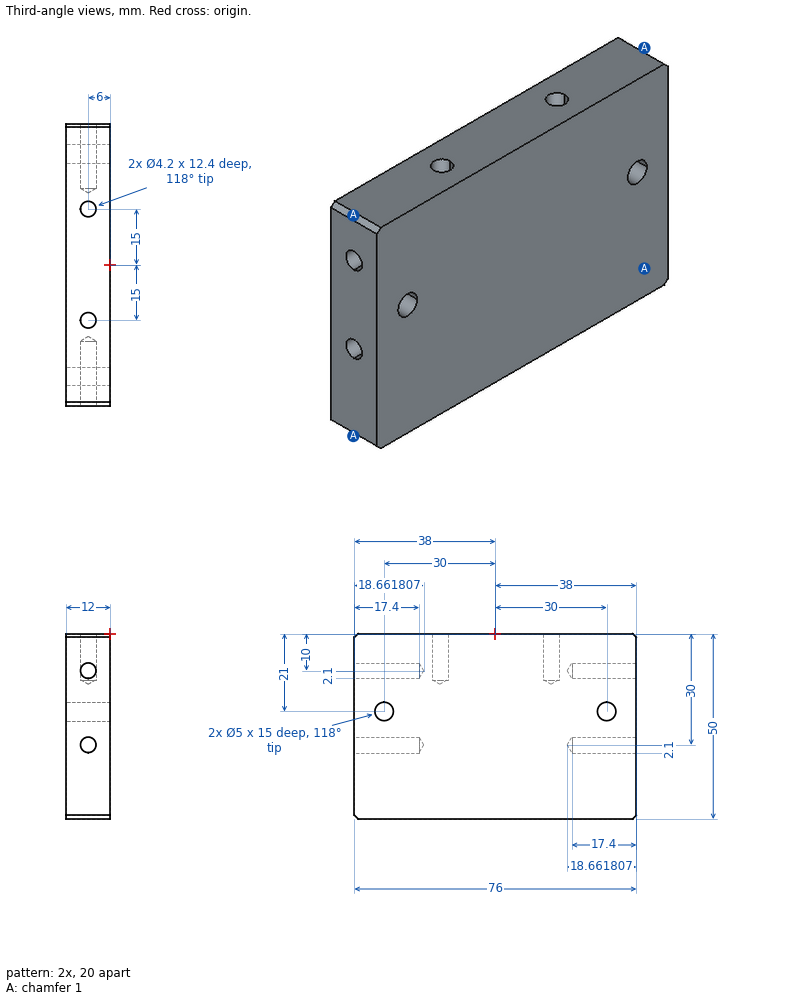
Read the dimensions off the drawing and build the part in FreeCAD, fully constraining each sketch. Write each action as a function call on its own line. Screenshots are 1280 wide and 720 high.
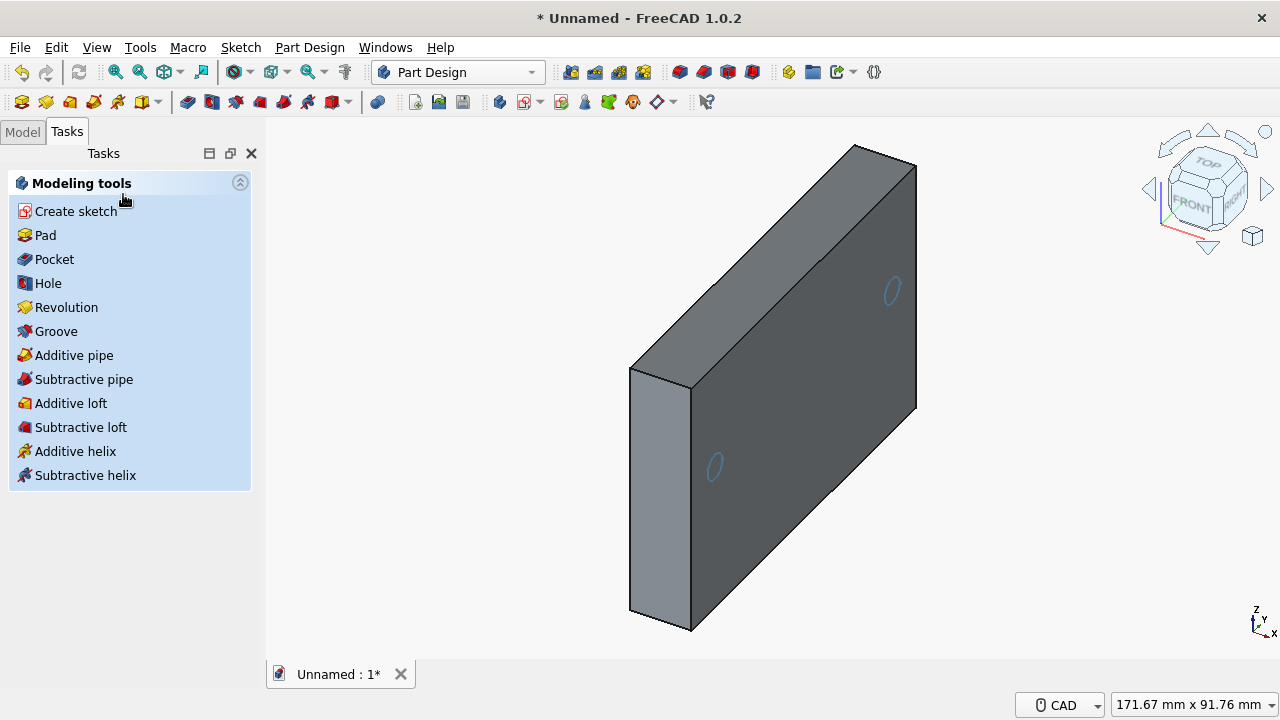
click(212, 102)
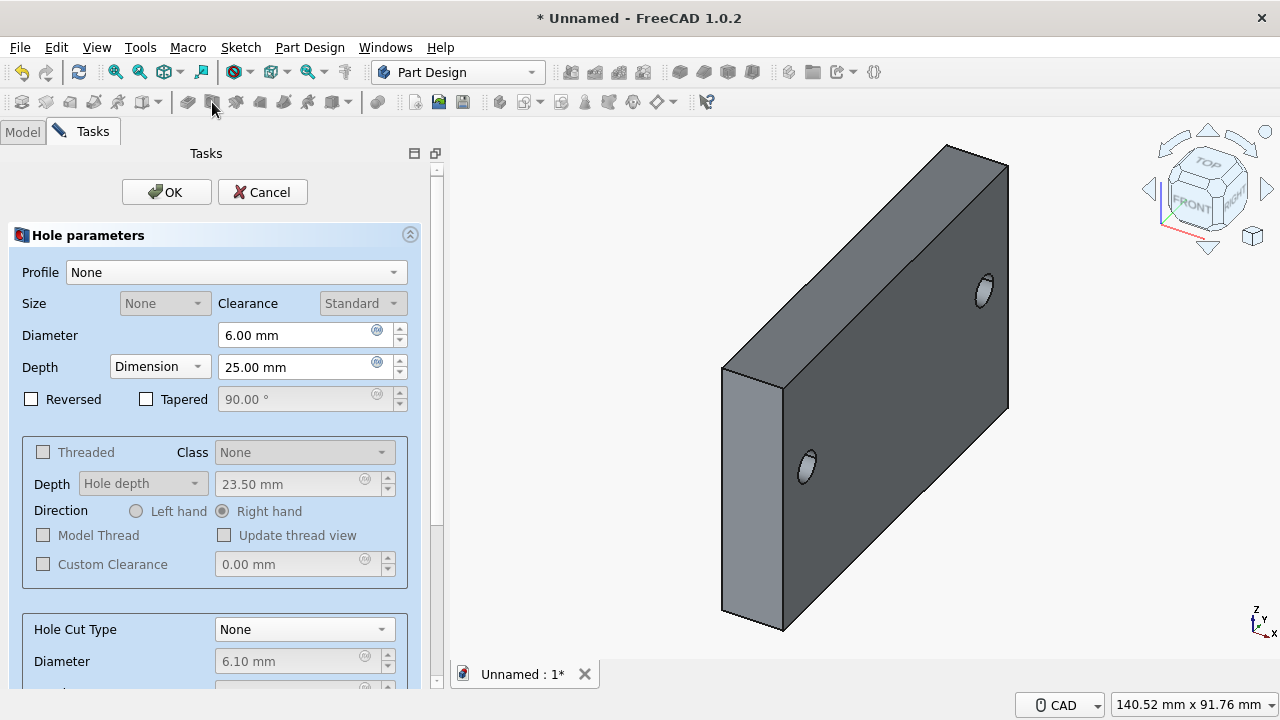
triple_click(305, 335)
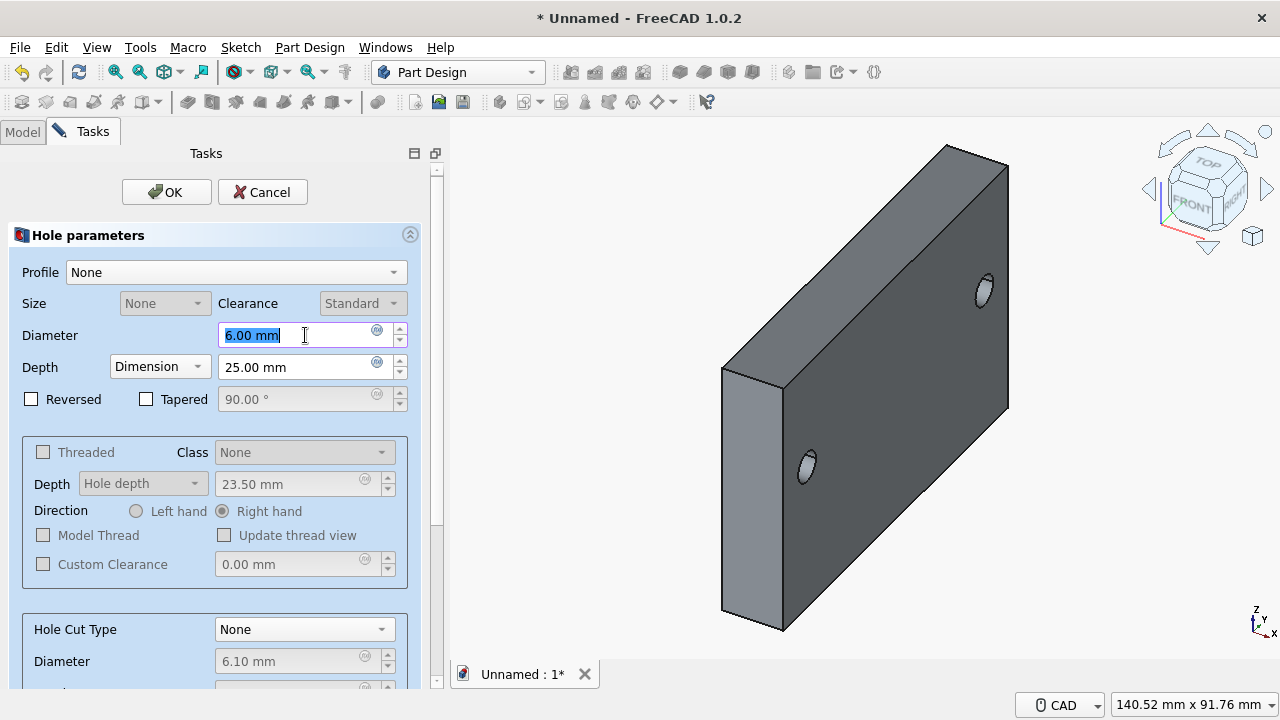
text(5)
key(Tab)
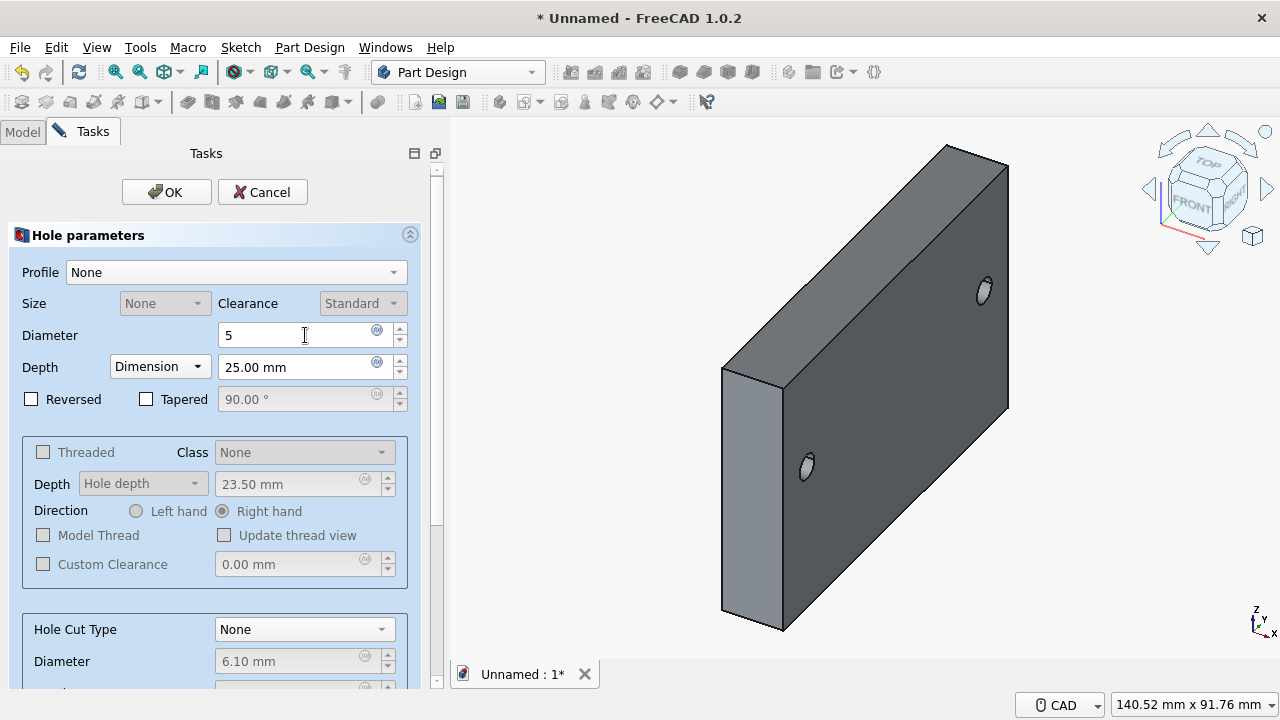
triple_click(305, 367)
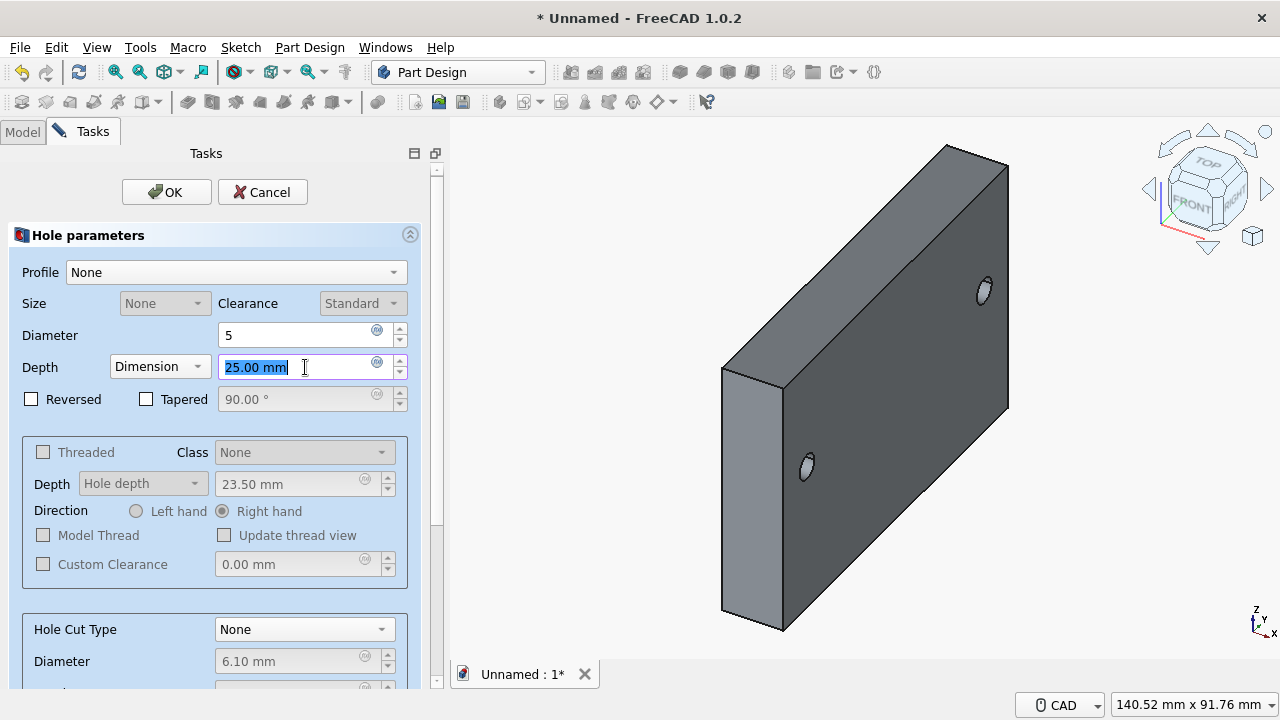
text(15)
key(Tab)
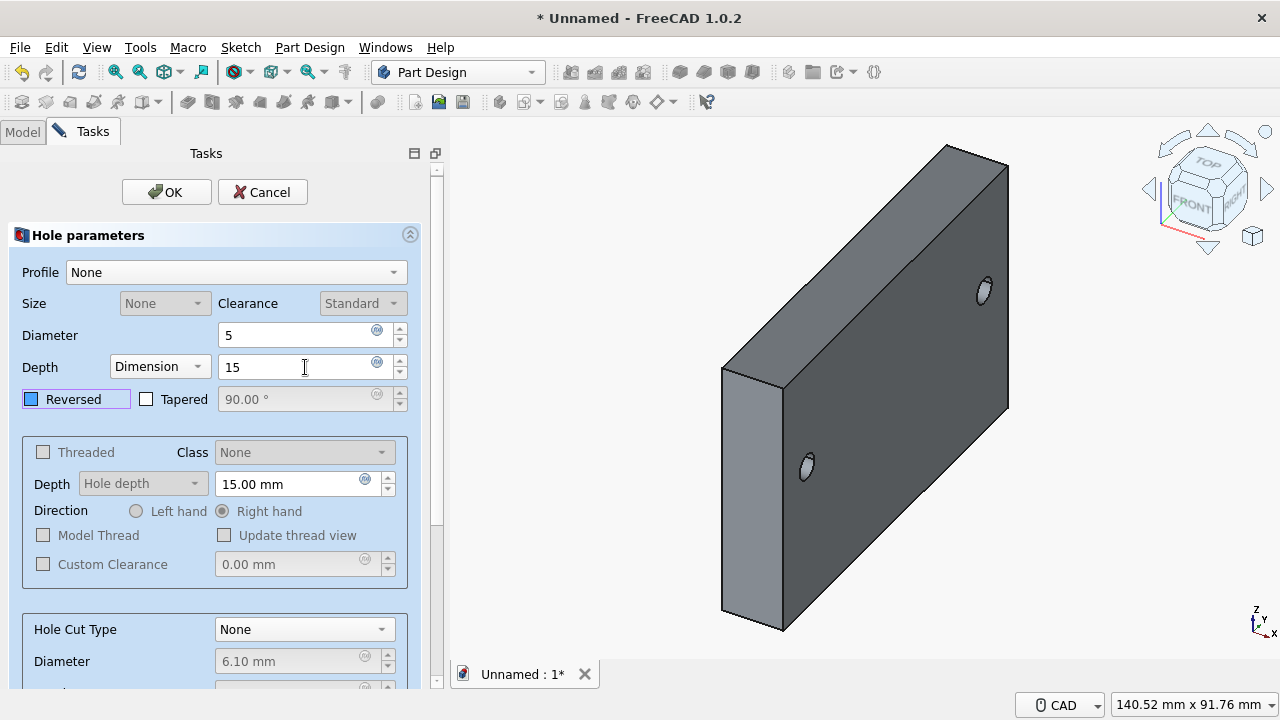
click(167, 192)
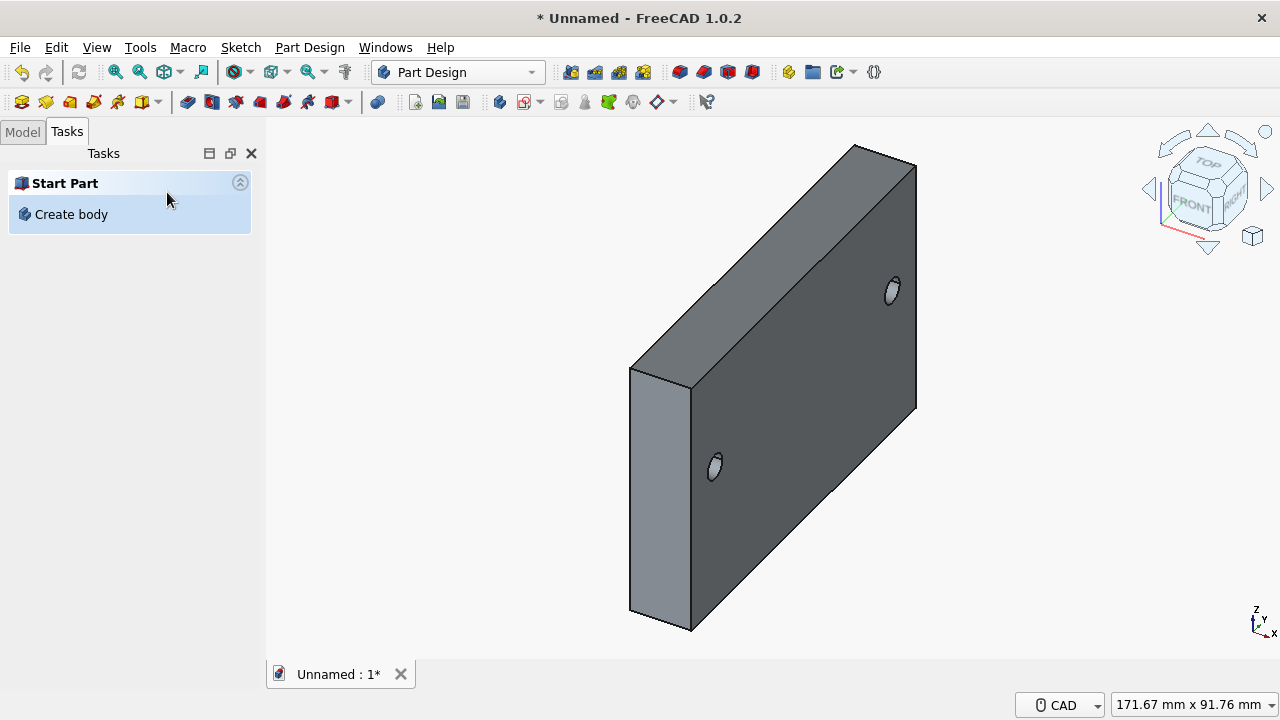
click(23, 131)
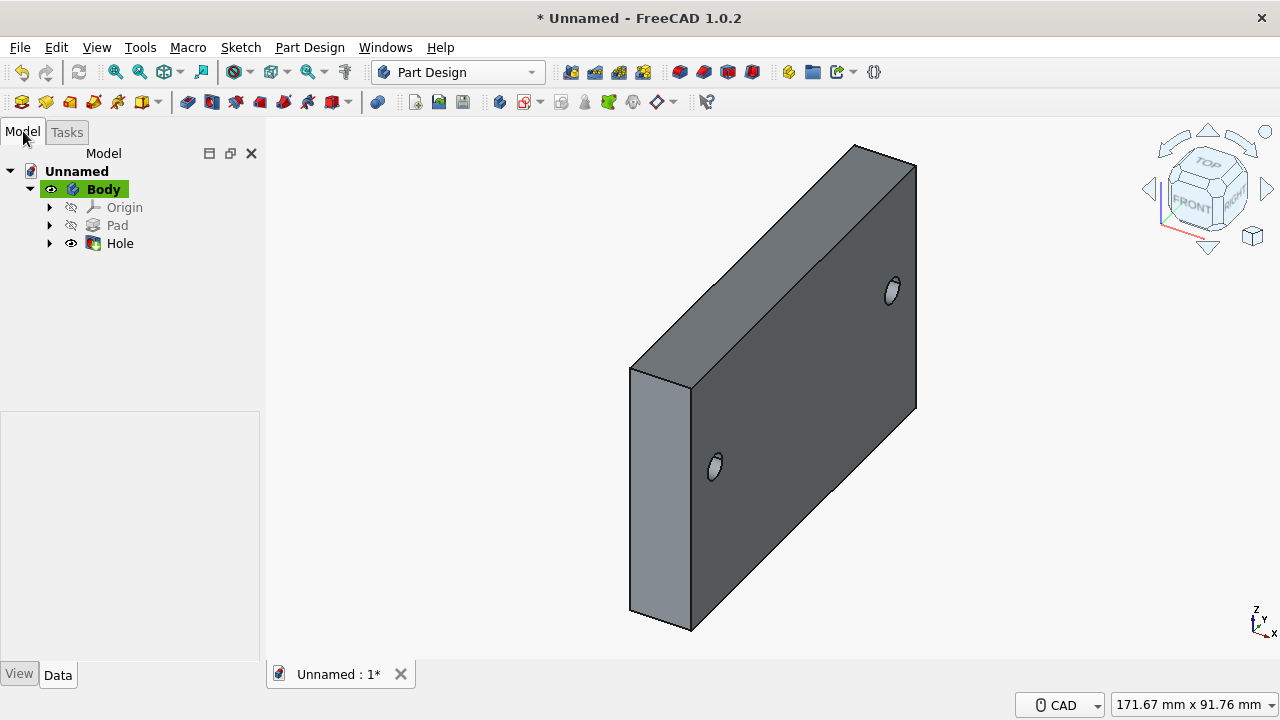
click(50, 207)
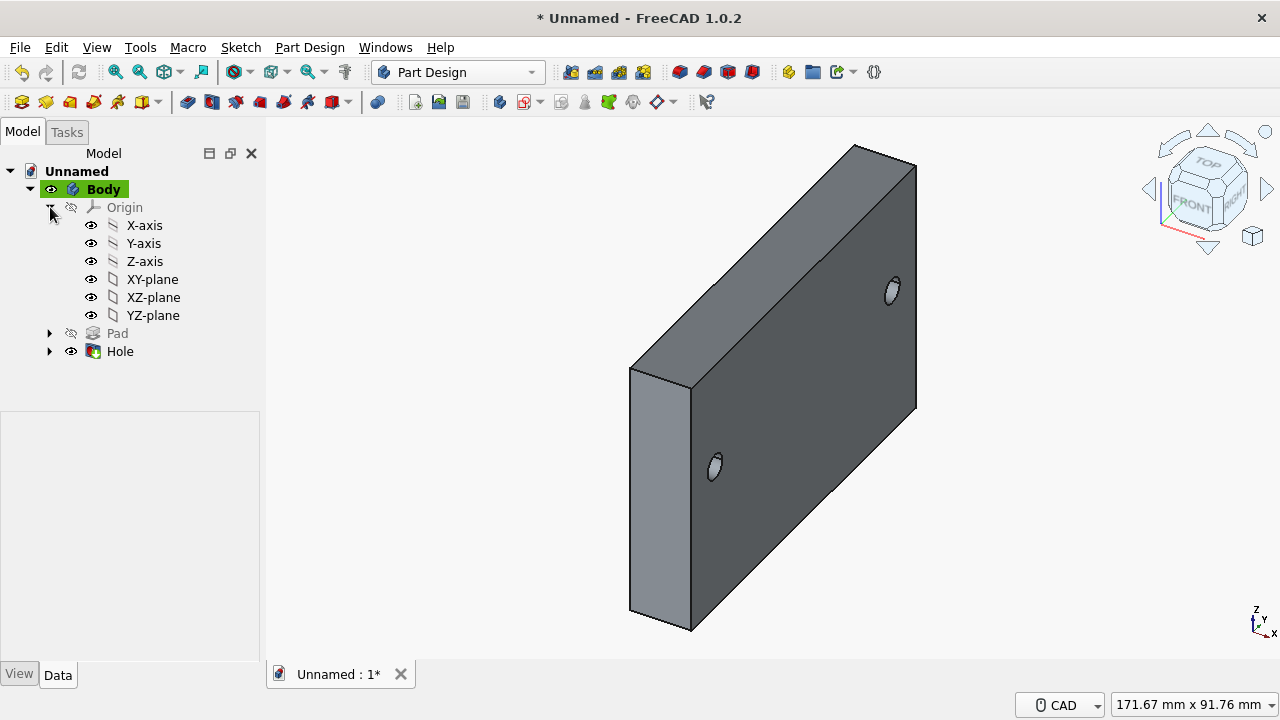
click(136, 315)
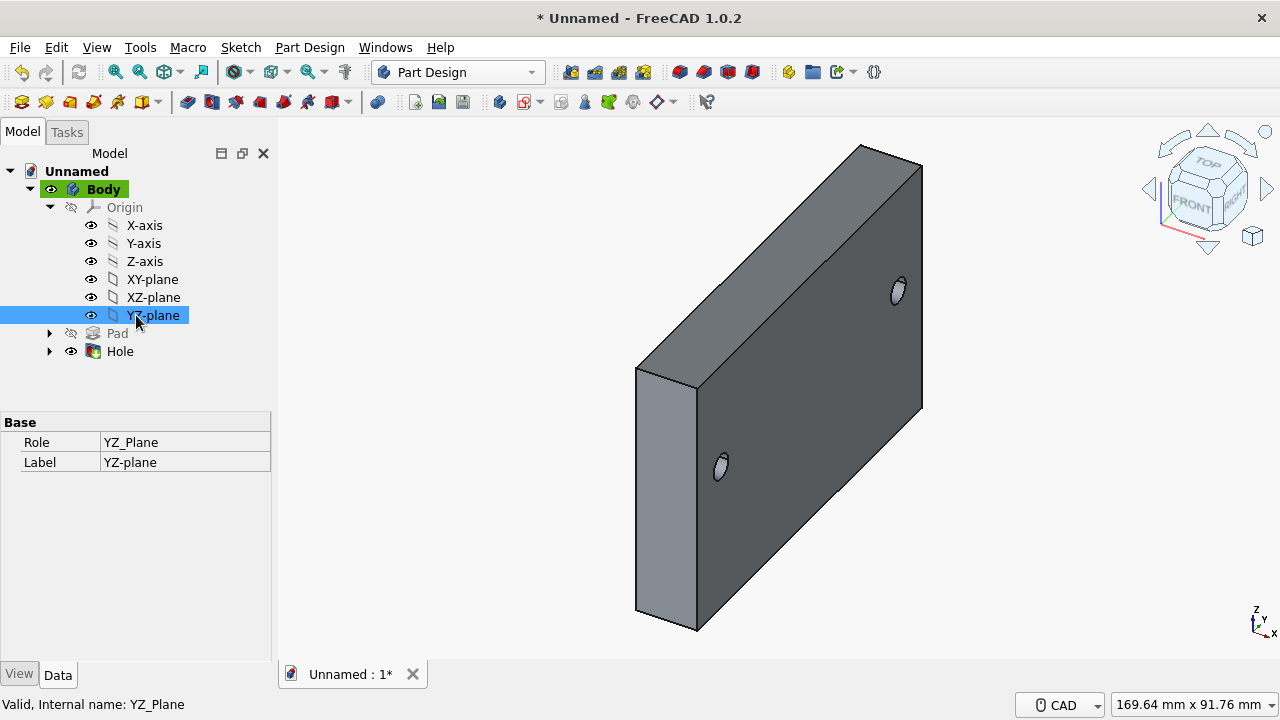
click(658, 102)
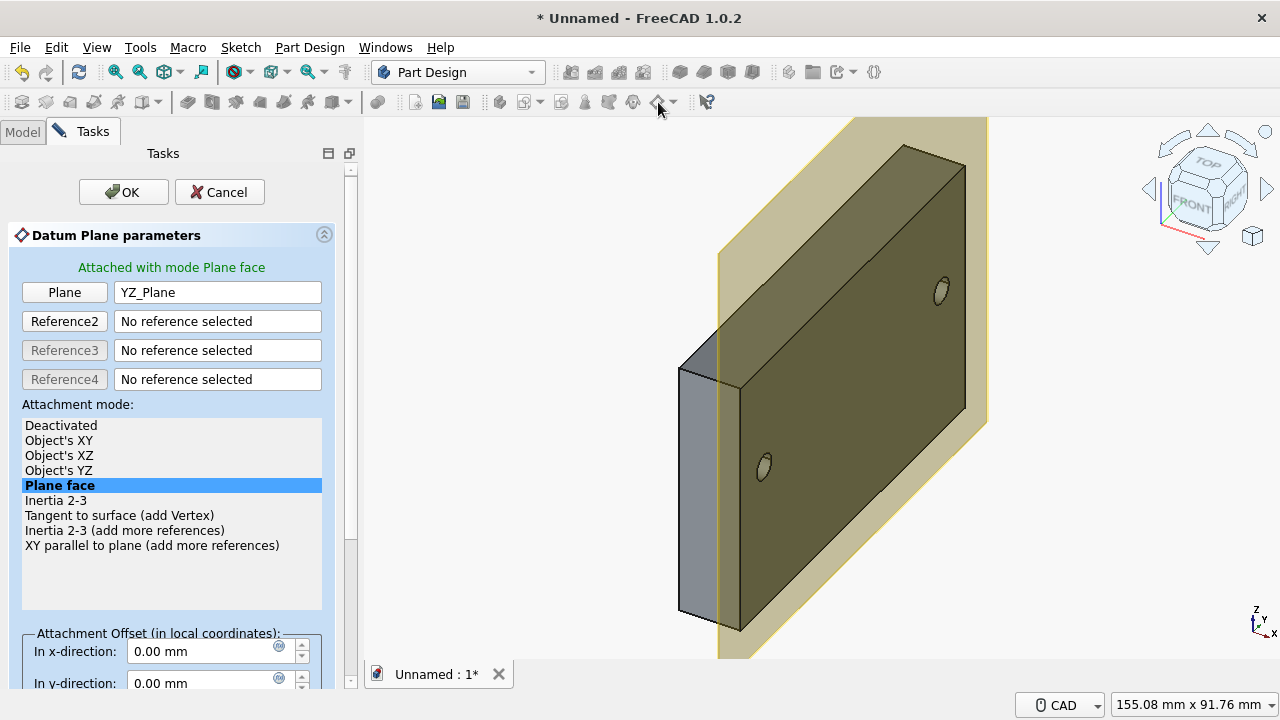
scroll(351, 426, down, 2)